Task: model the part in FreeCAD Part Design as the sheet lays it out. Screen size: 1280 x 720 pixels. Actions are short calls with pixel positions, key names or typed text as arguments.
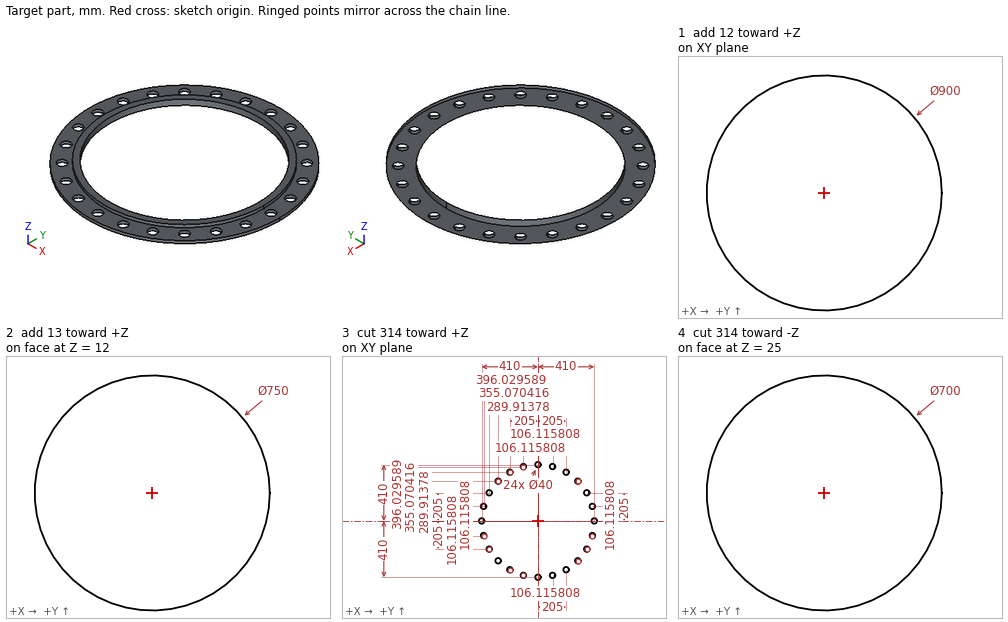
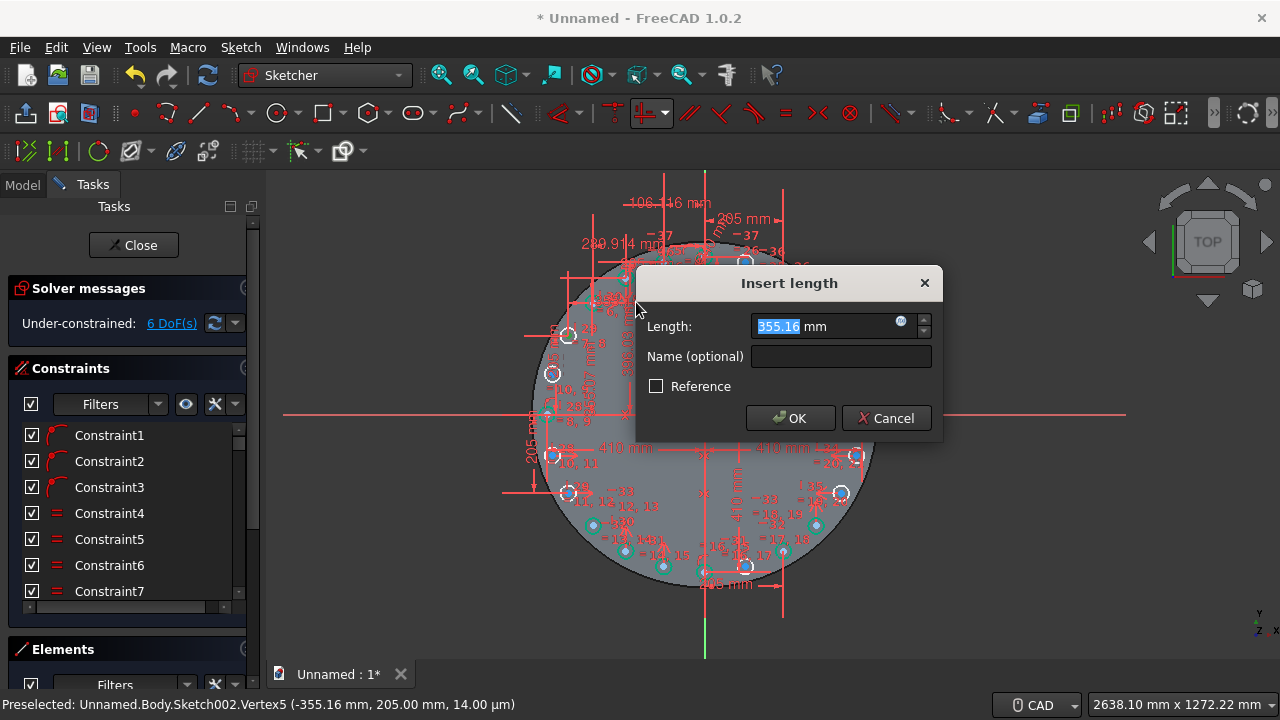
text(355.070416)
key(Return)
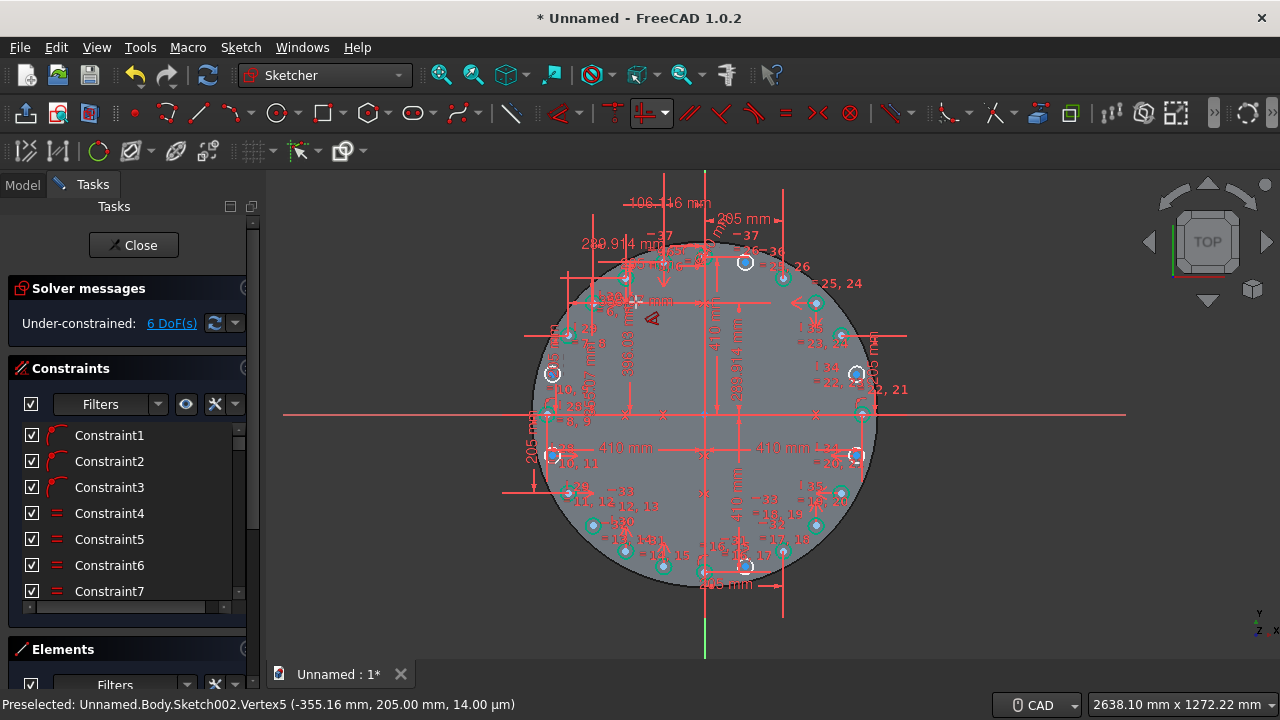
click(553, 374)
click(629, 473)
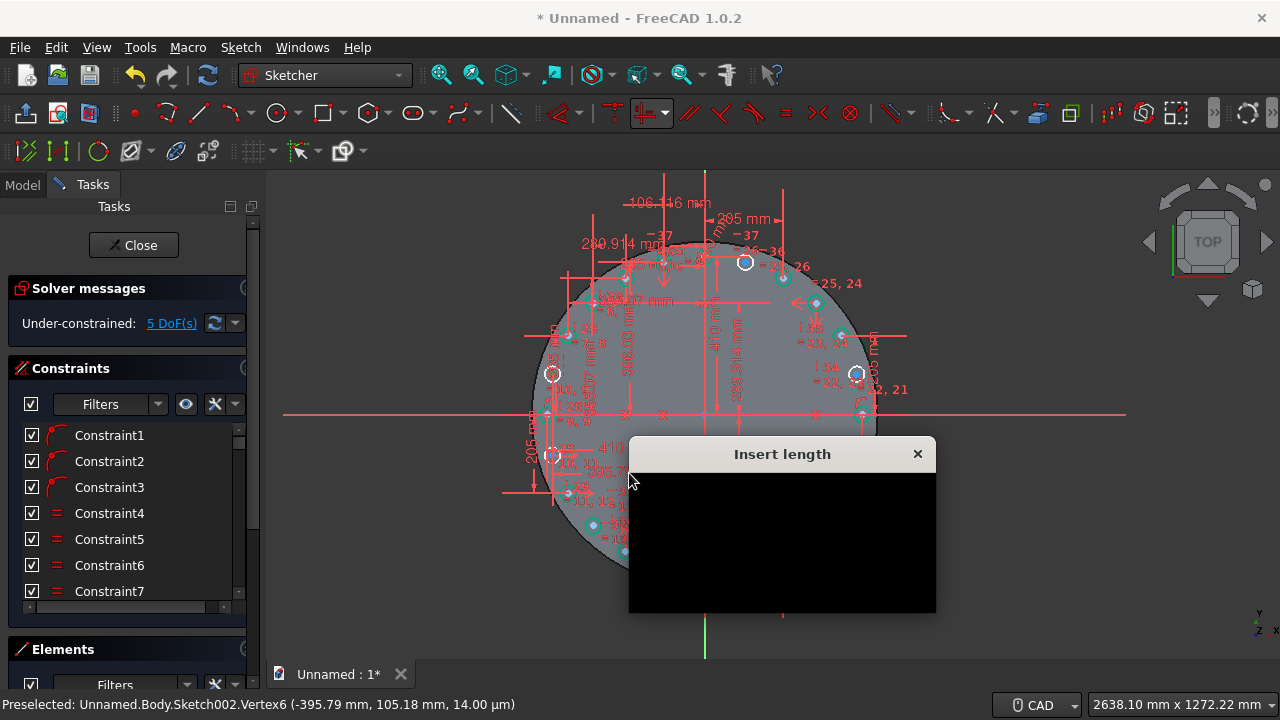
text(396.029589)
key(Return)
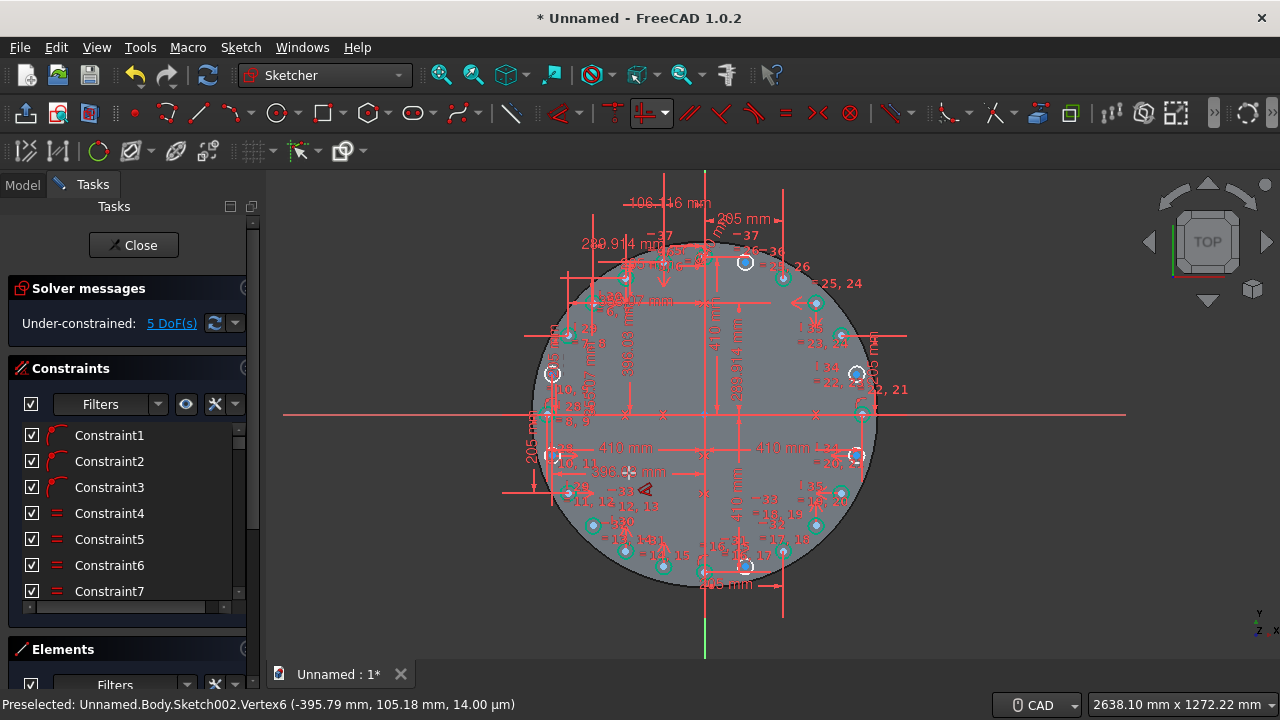
click(552, 374)
click(518, 394)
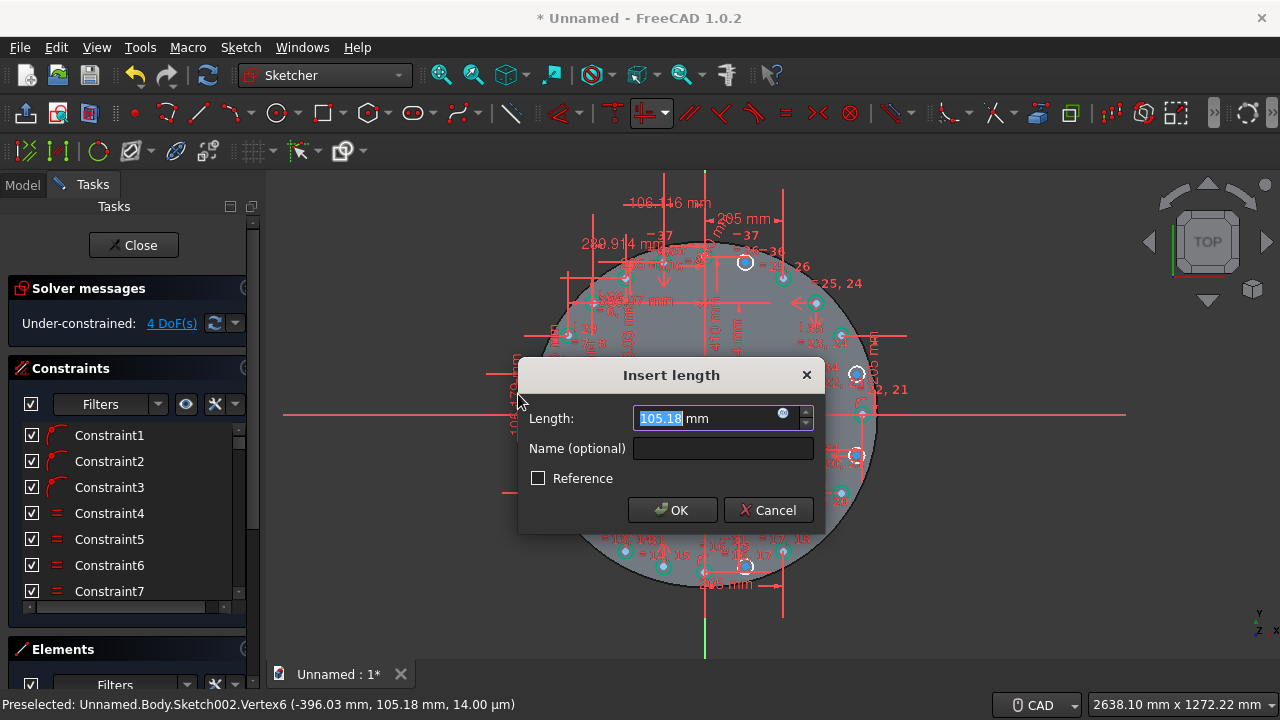
text(106.115808)
key(Return)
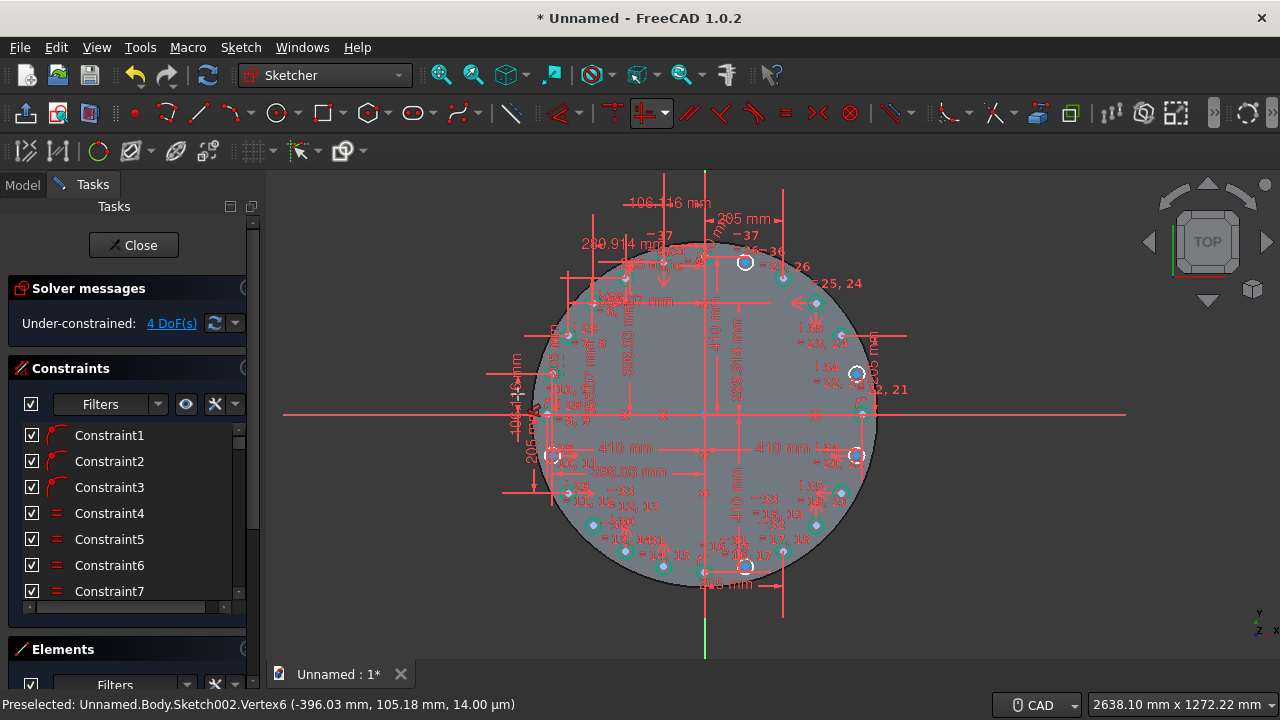
click(552, 456)
click(446, 435)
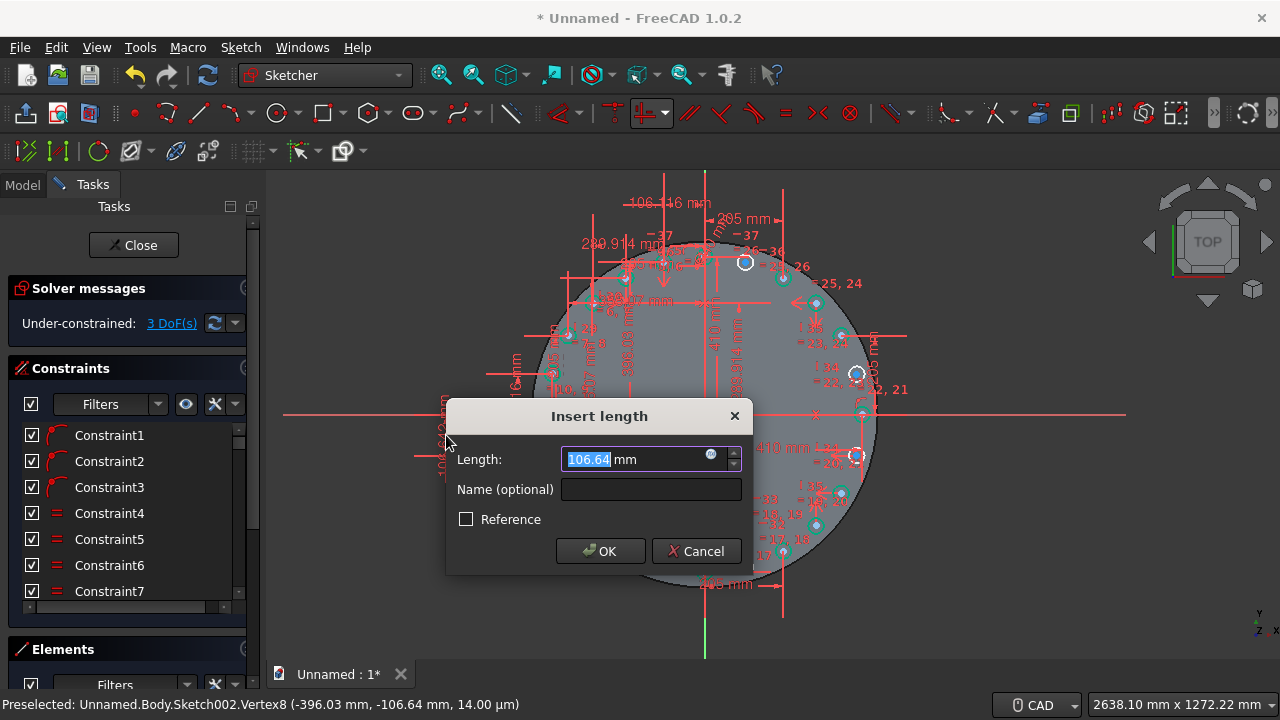
text(106.115808)
key(Return)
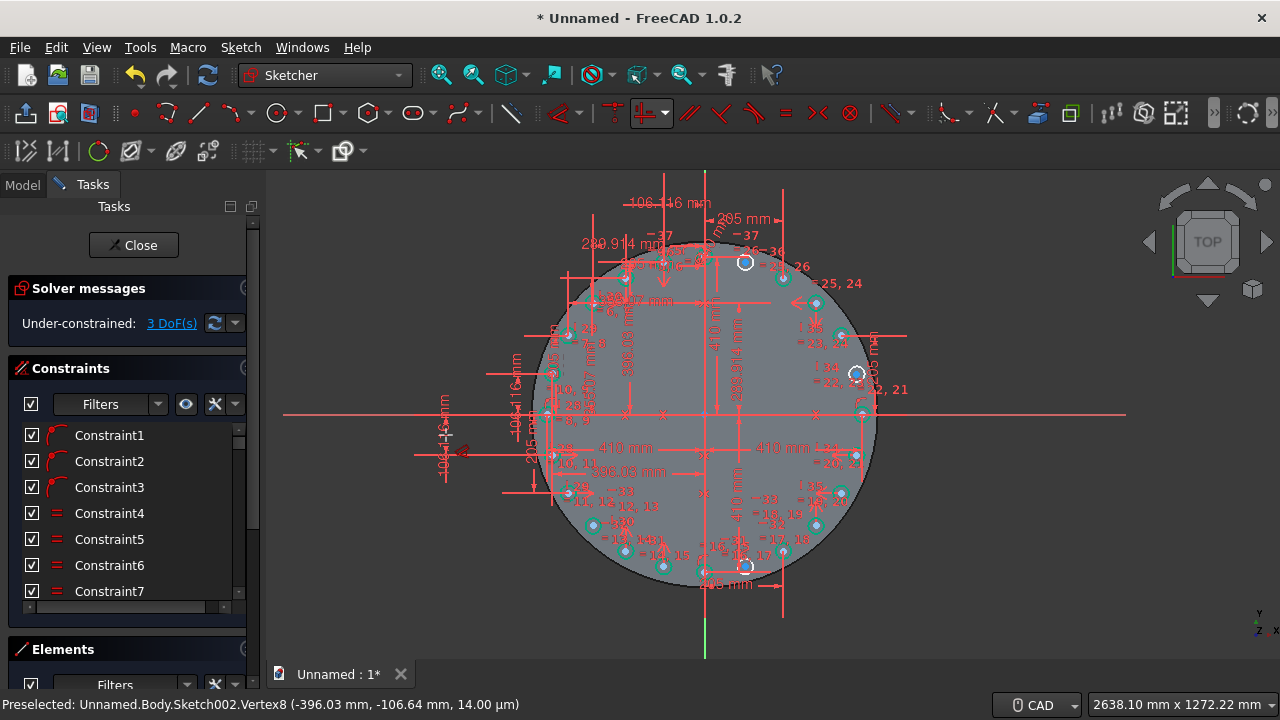
click(745, 567)
click(725, 381)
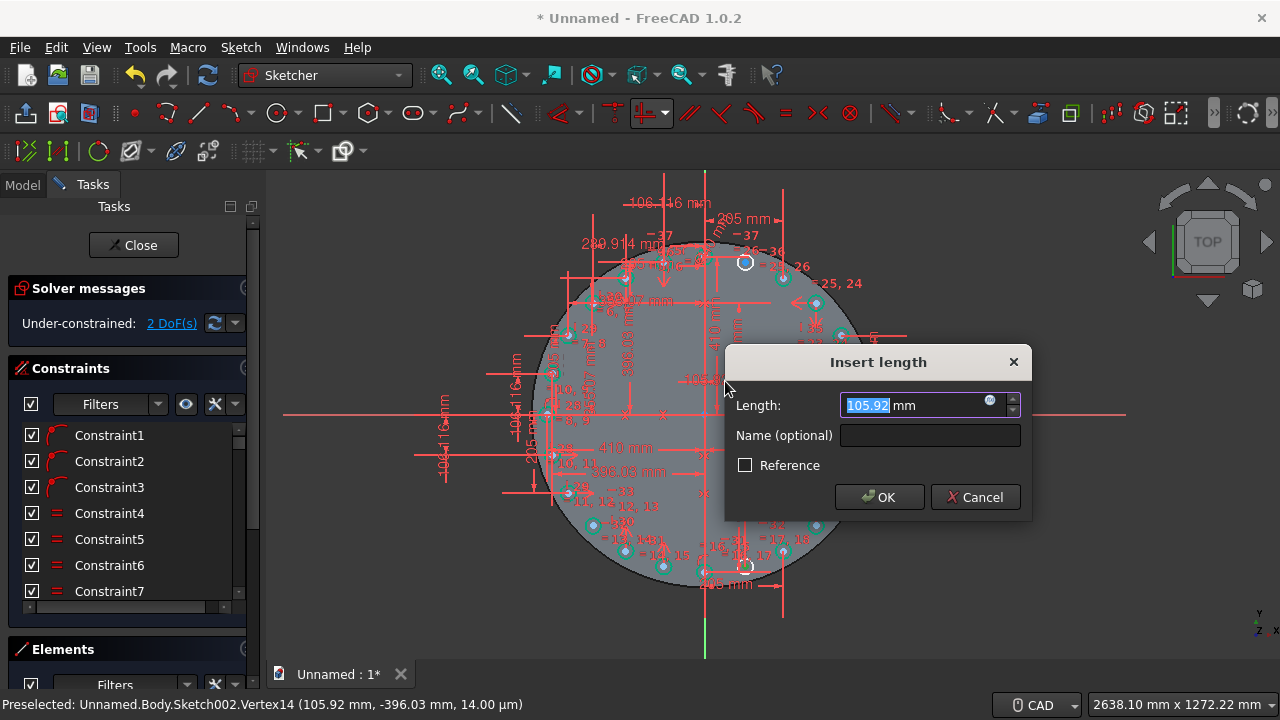
text(106.115808)
key(Return)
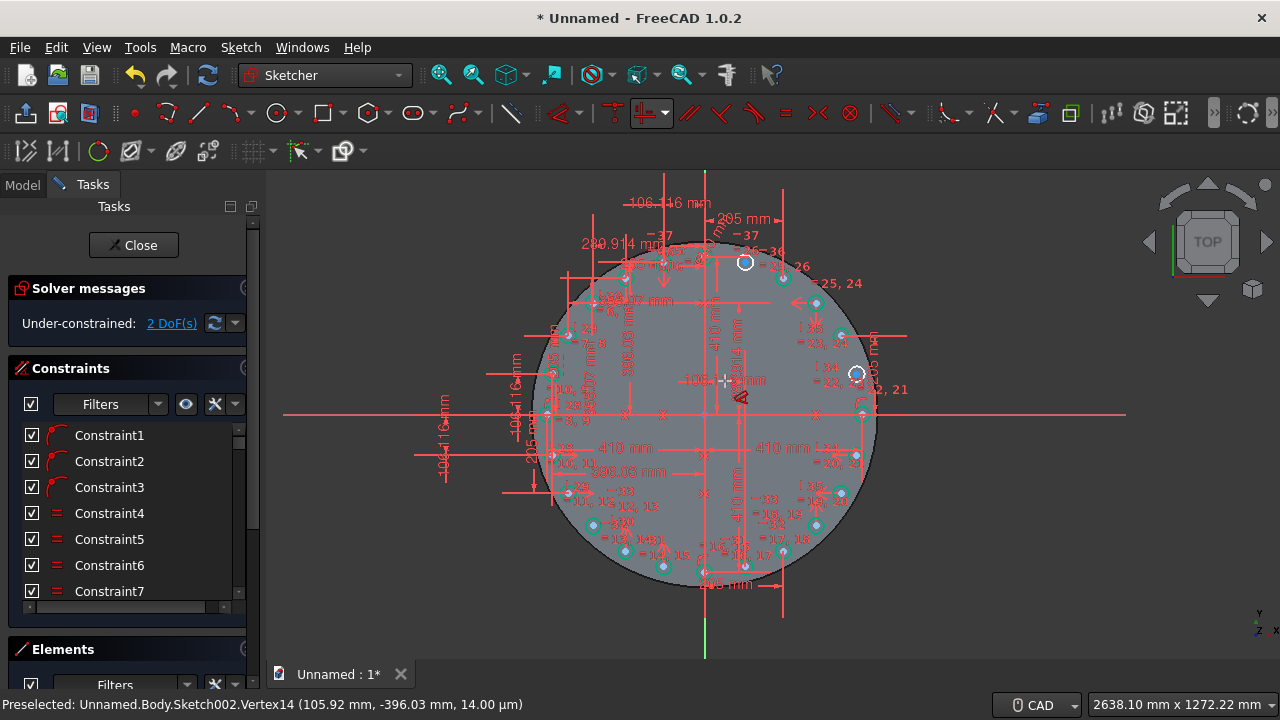
click(857, 374)
click(891, 394)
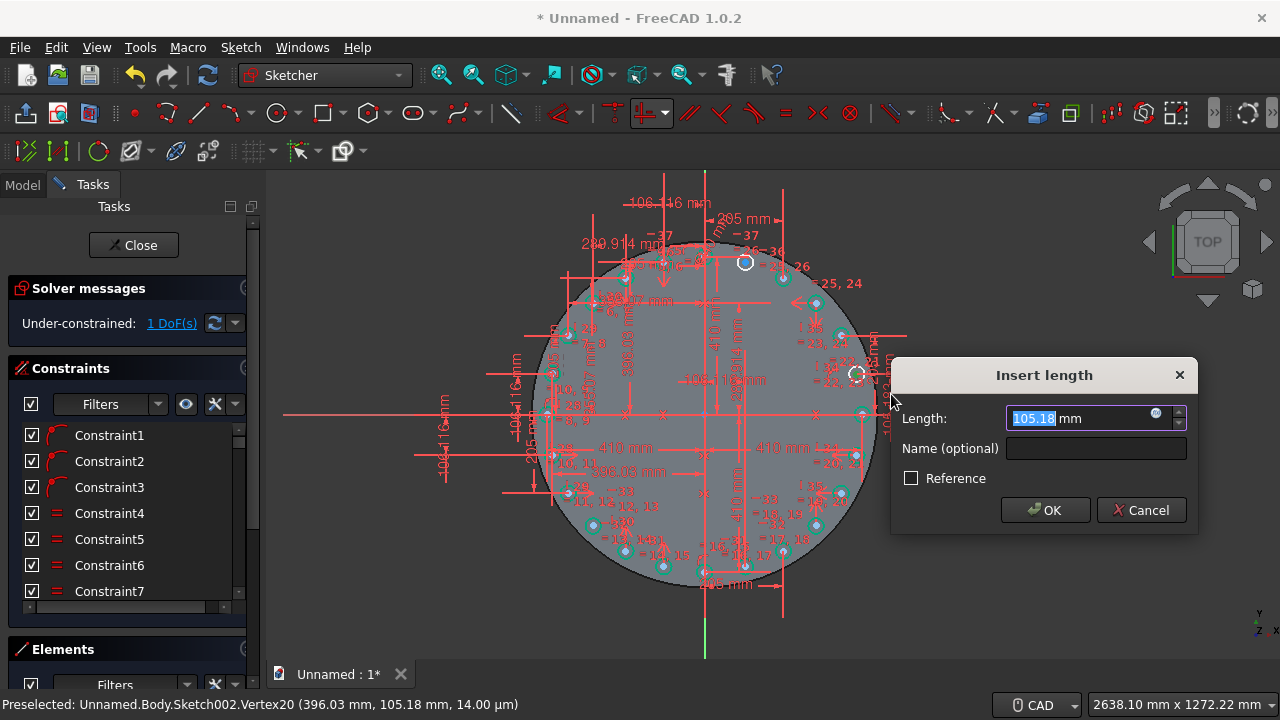
text(106.115808)
key(Return)